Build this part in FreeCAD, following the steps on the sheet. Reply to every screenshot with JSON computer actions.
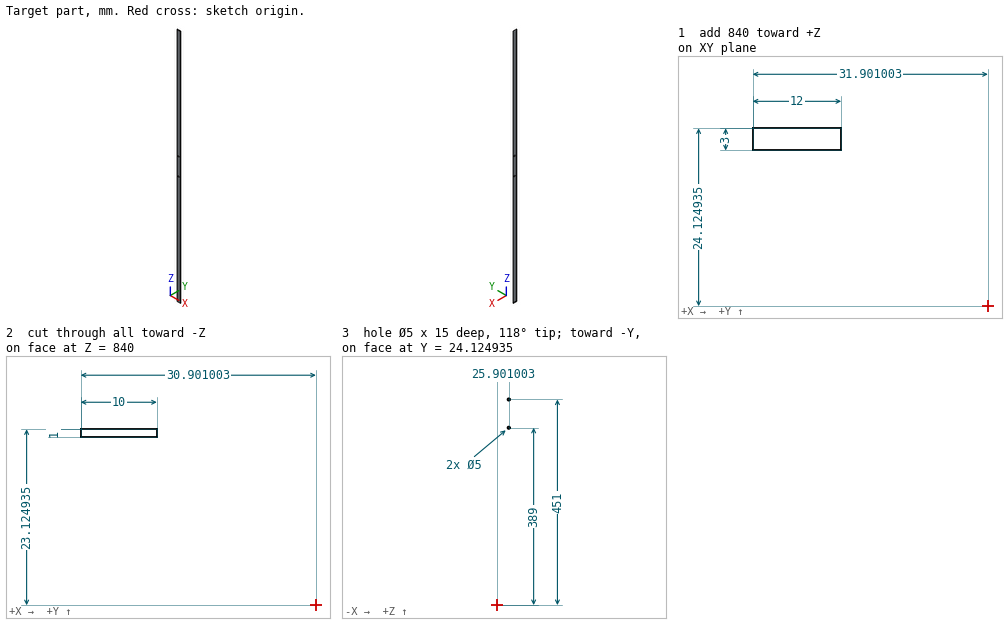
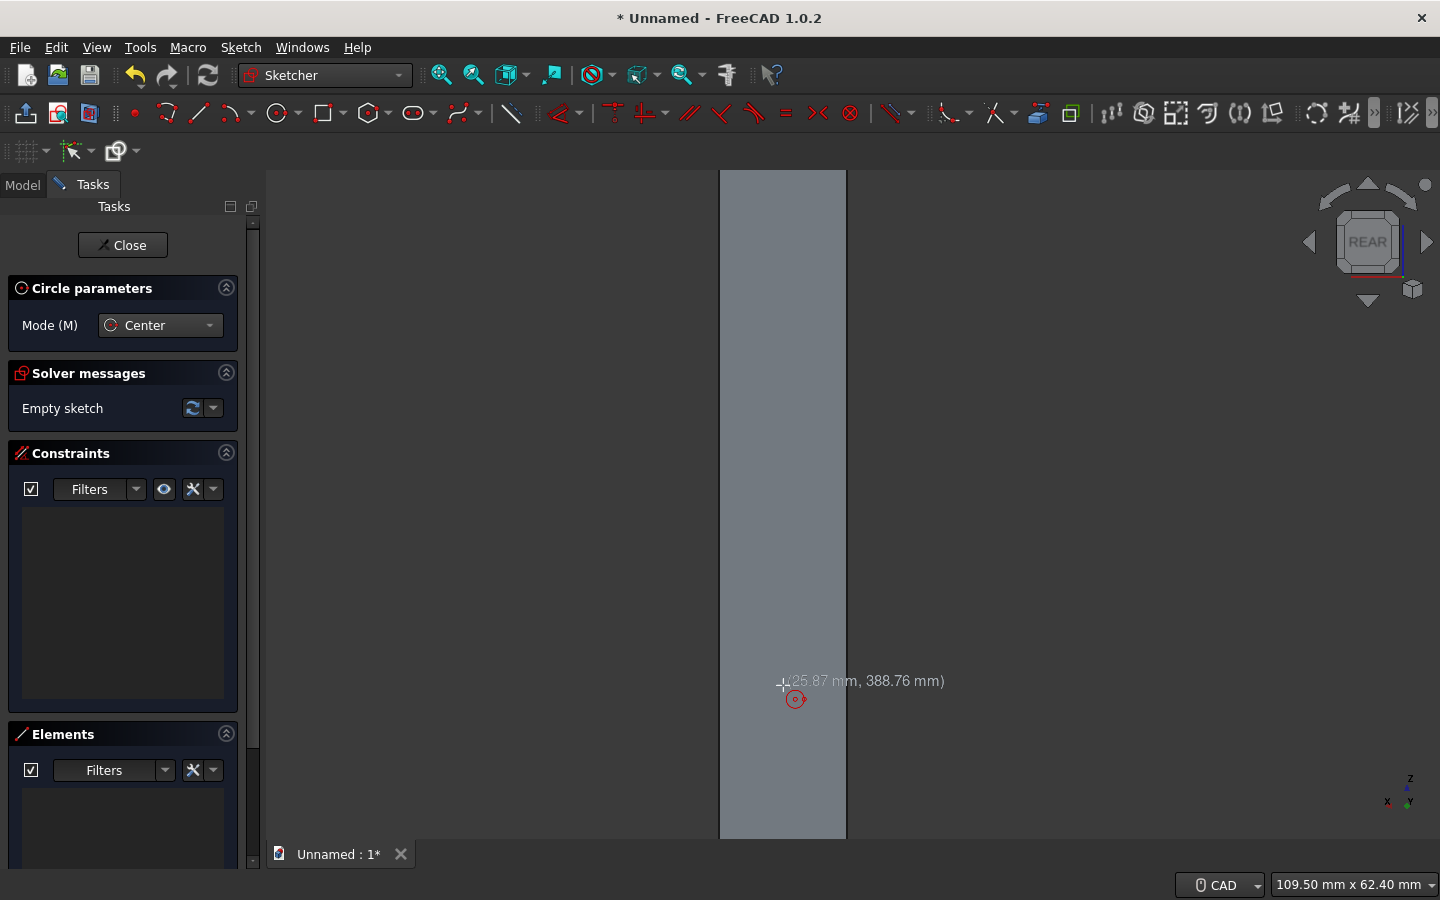
{"action": "left_click", "coordinate": [783, 684]}
{"action": "mouse_move", "coordinate": [802, 665]}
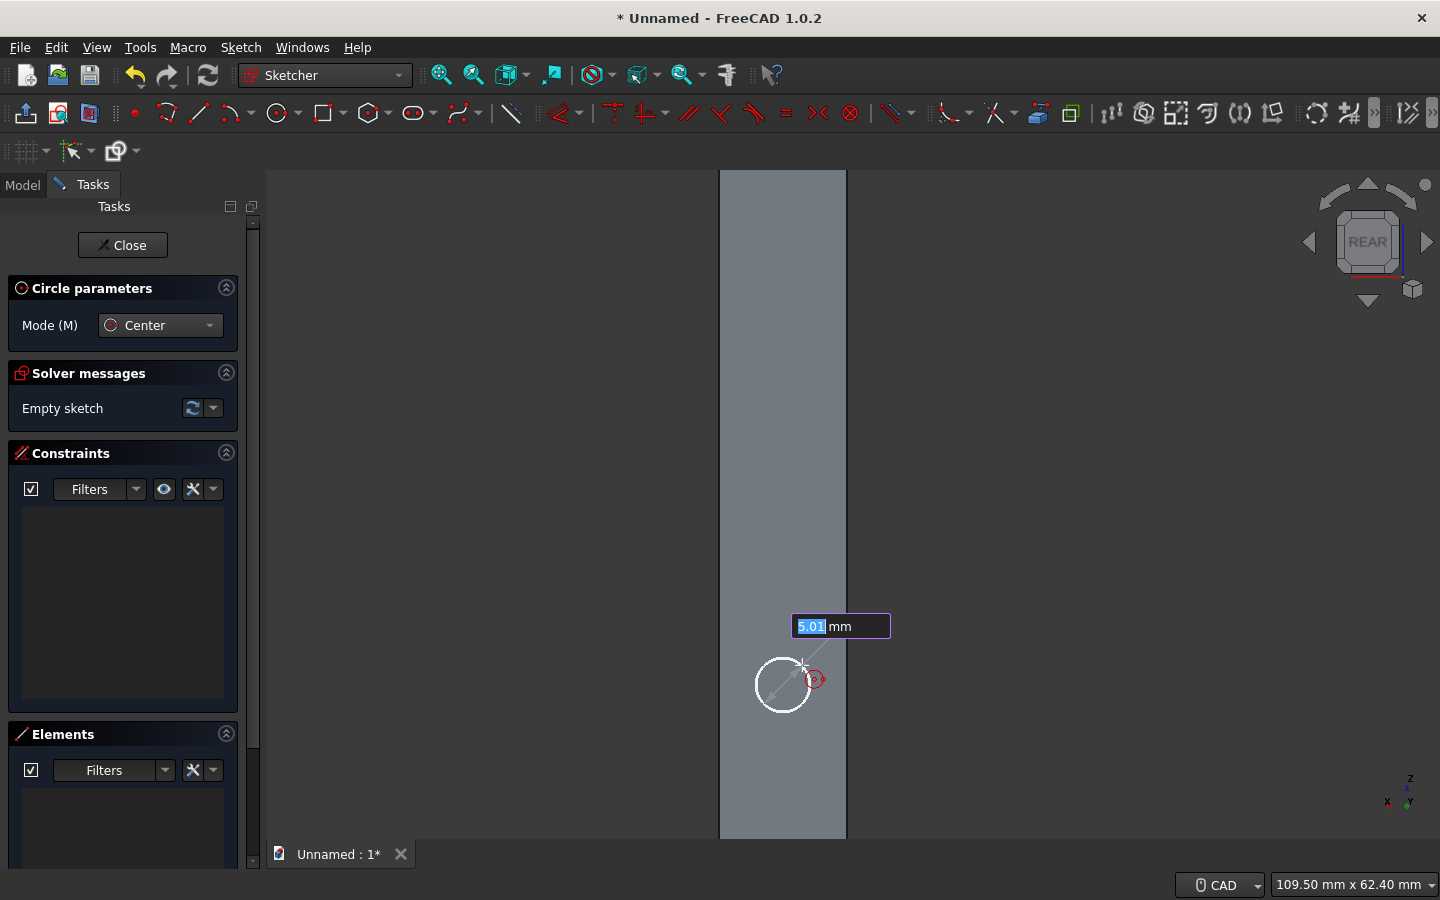
{"action": "type", "text": "5"}
{"action": "key", "text": "Return"}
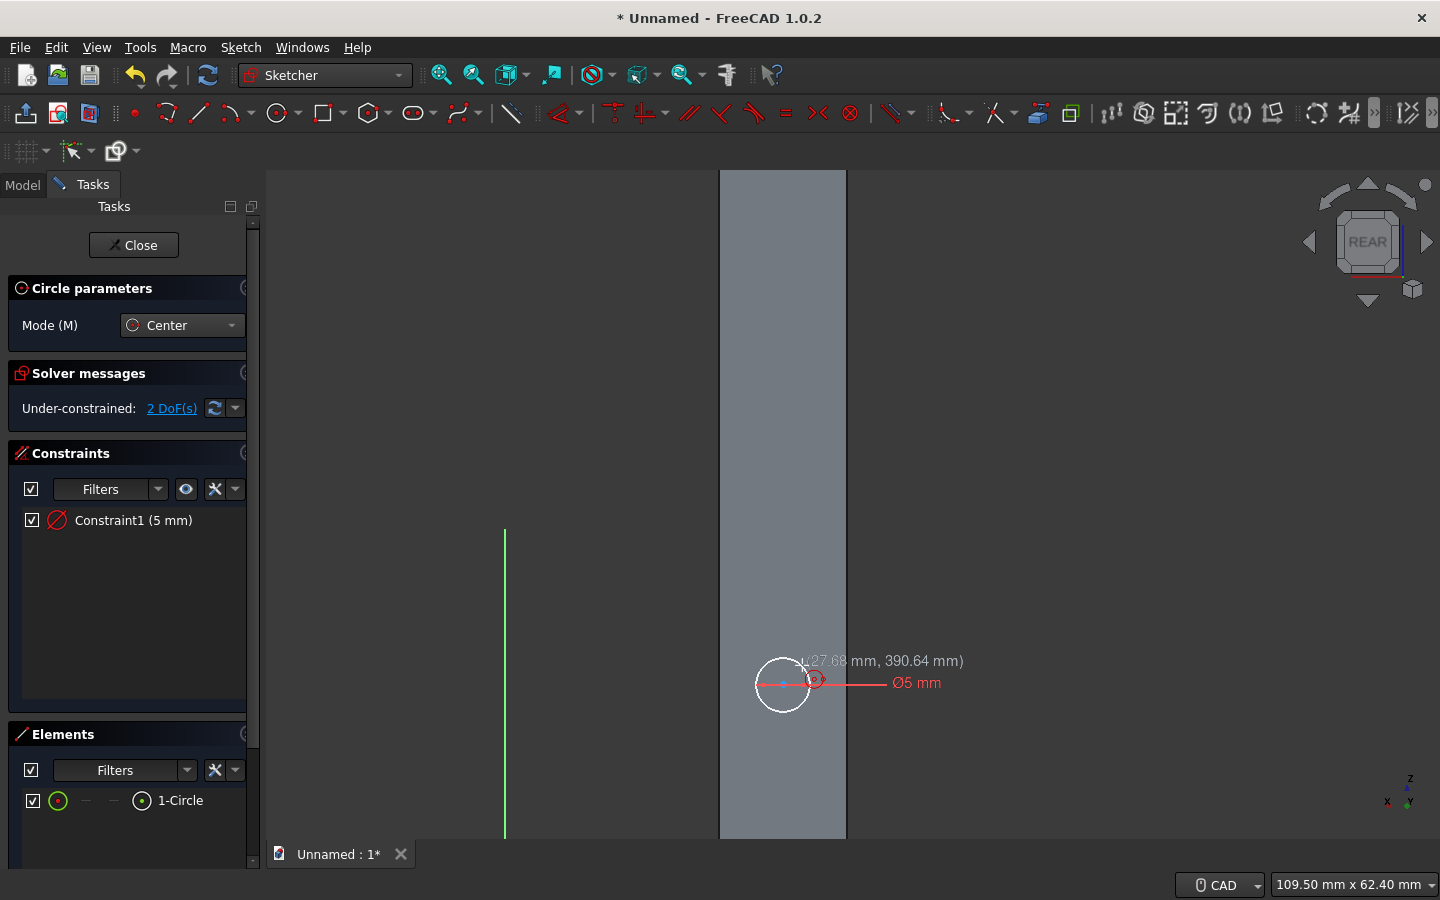
{"action": "scroll", "coordinate": [786, 691], "scroll_direction": "down", "scroll_amount": 3}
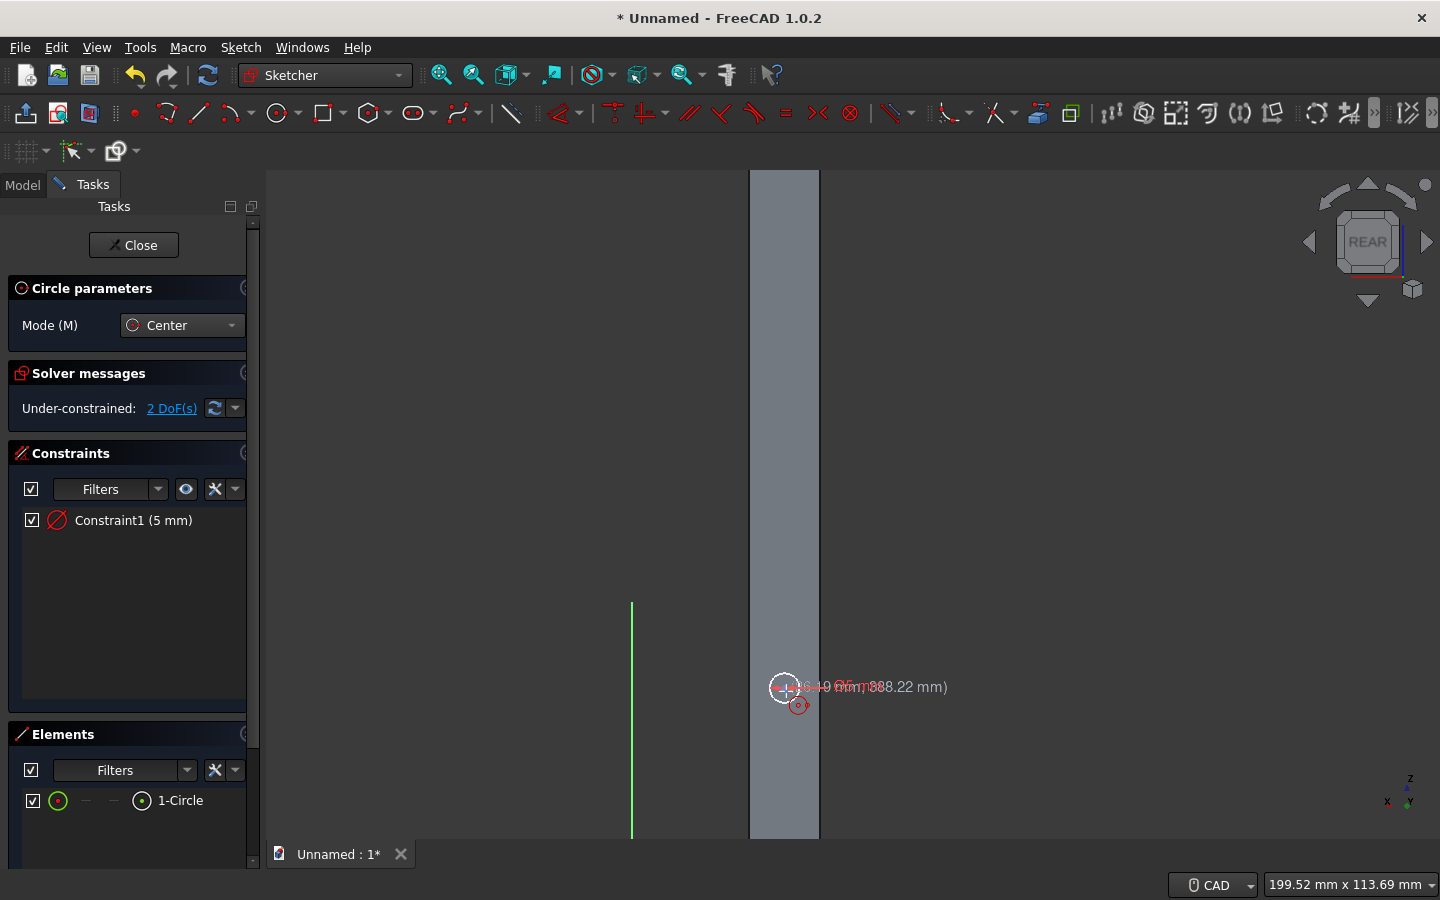
{"action": "scroll", "coordinate": [785, 322], "scroll_direction": "up", "scroll_amount": 3}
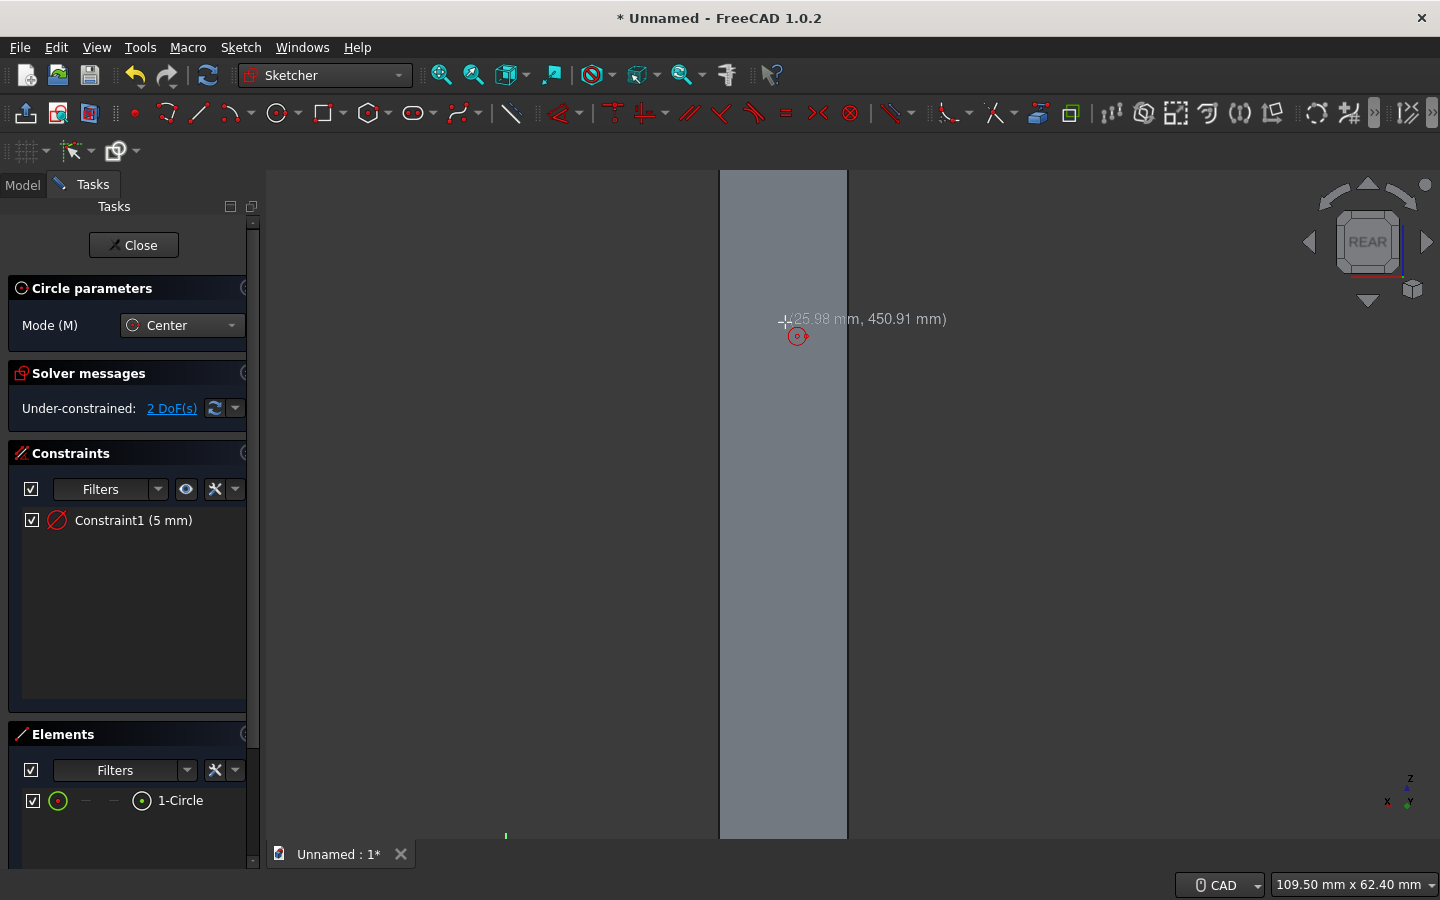
{"action": "left_click", "coordinate": [784, 323]}
{"action": "mouse_move", "coordinate": [803, 304]}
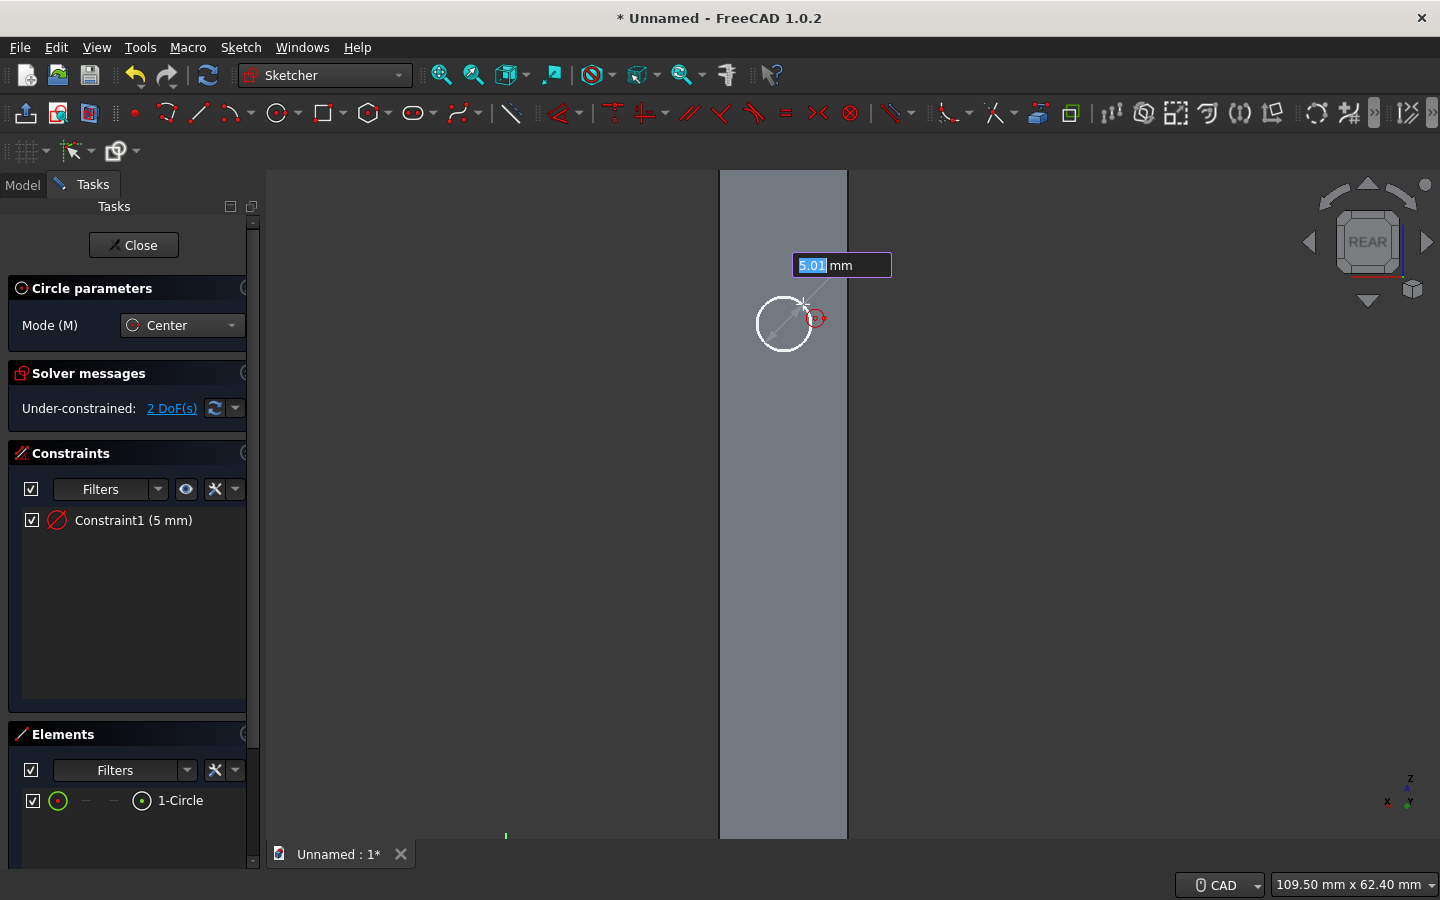
{"action": "type", "text": "5"}
{"action": "key", "text": "Return"}
{"action": "key", "text": "Escape"}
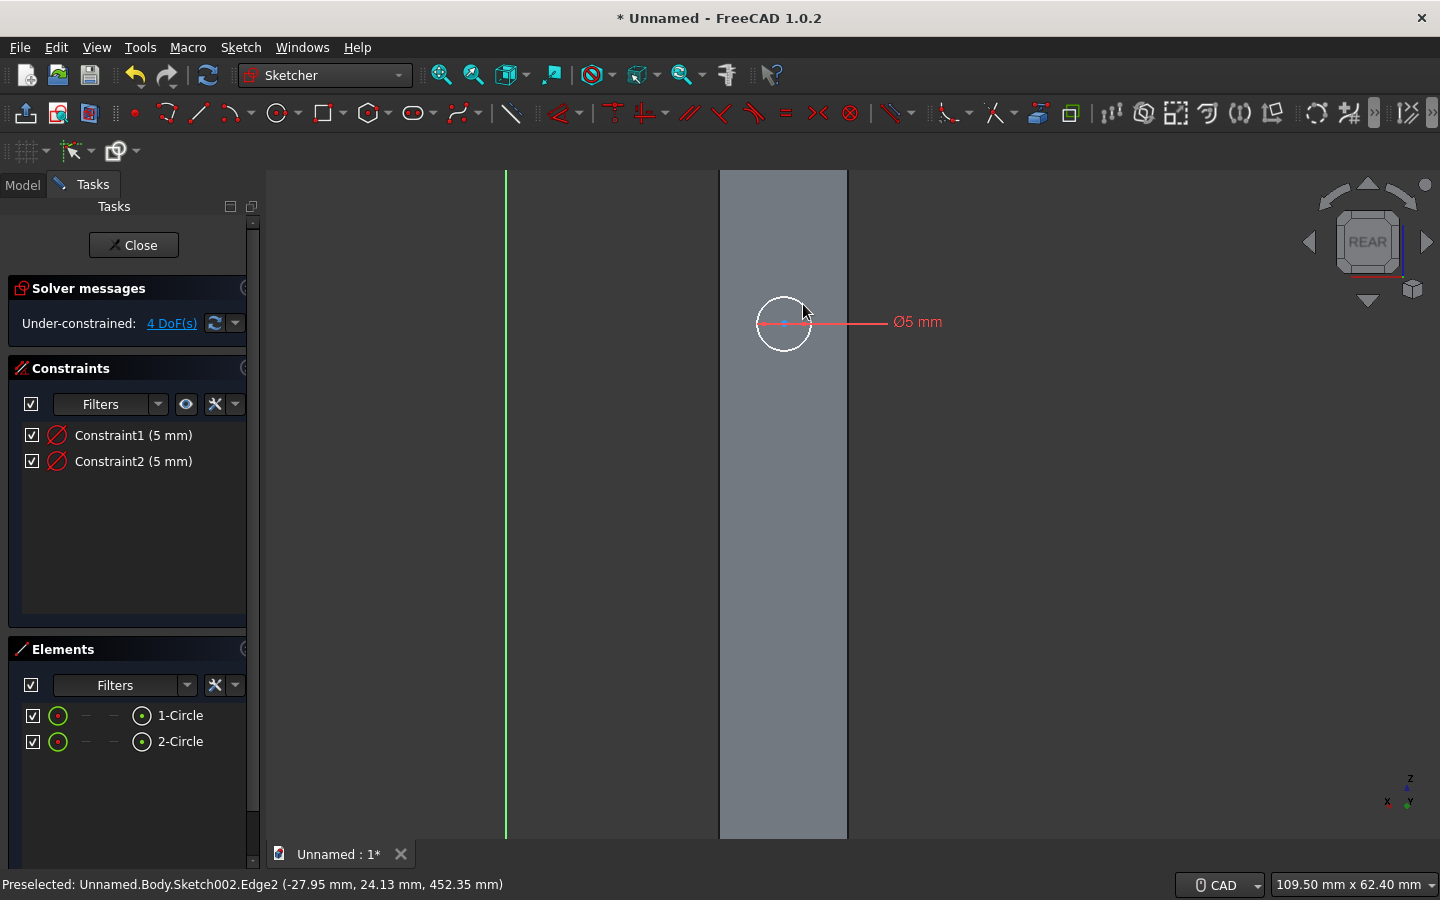
{"action": "scroll", "coordinate": [785, 321], "scroll_direction": "down", "scroll_amount": 3}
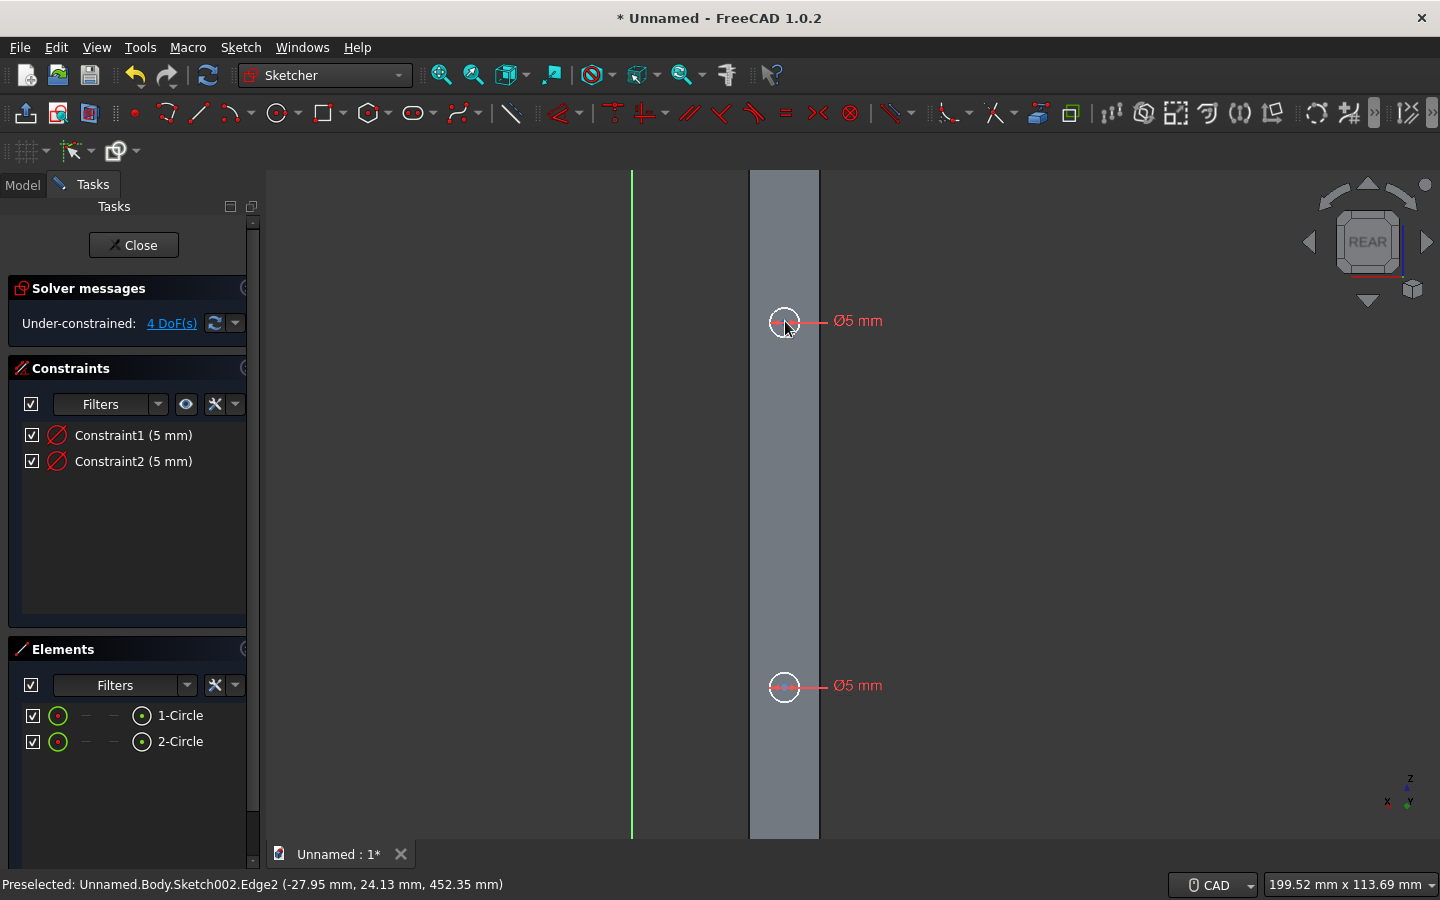
{"action": "left_click", "coordinate": [785, 688]}